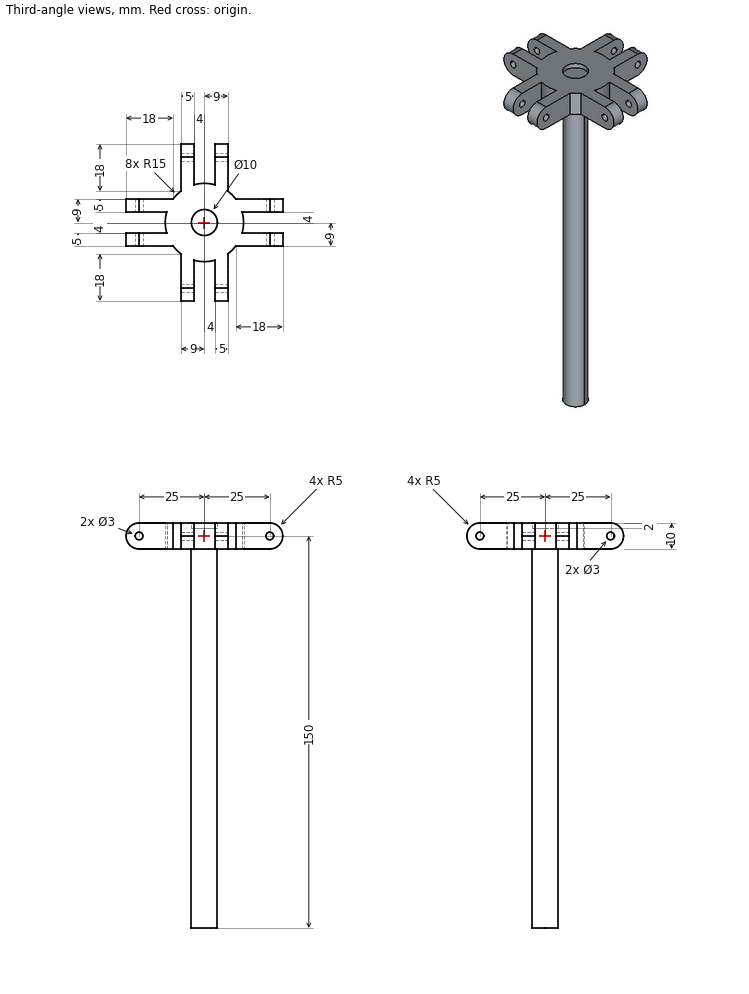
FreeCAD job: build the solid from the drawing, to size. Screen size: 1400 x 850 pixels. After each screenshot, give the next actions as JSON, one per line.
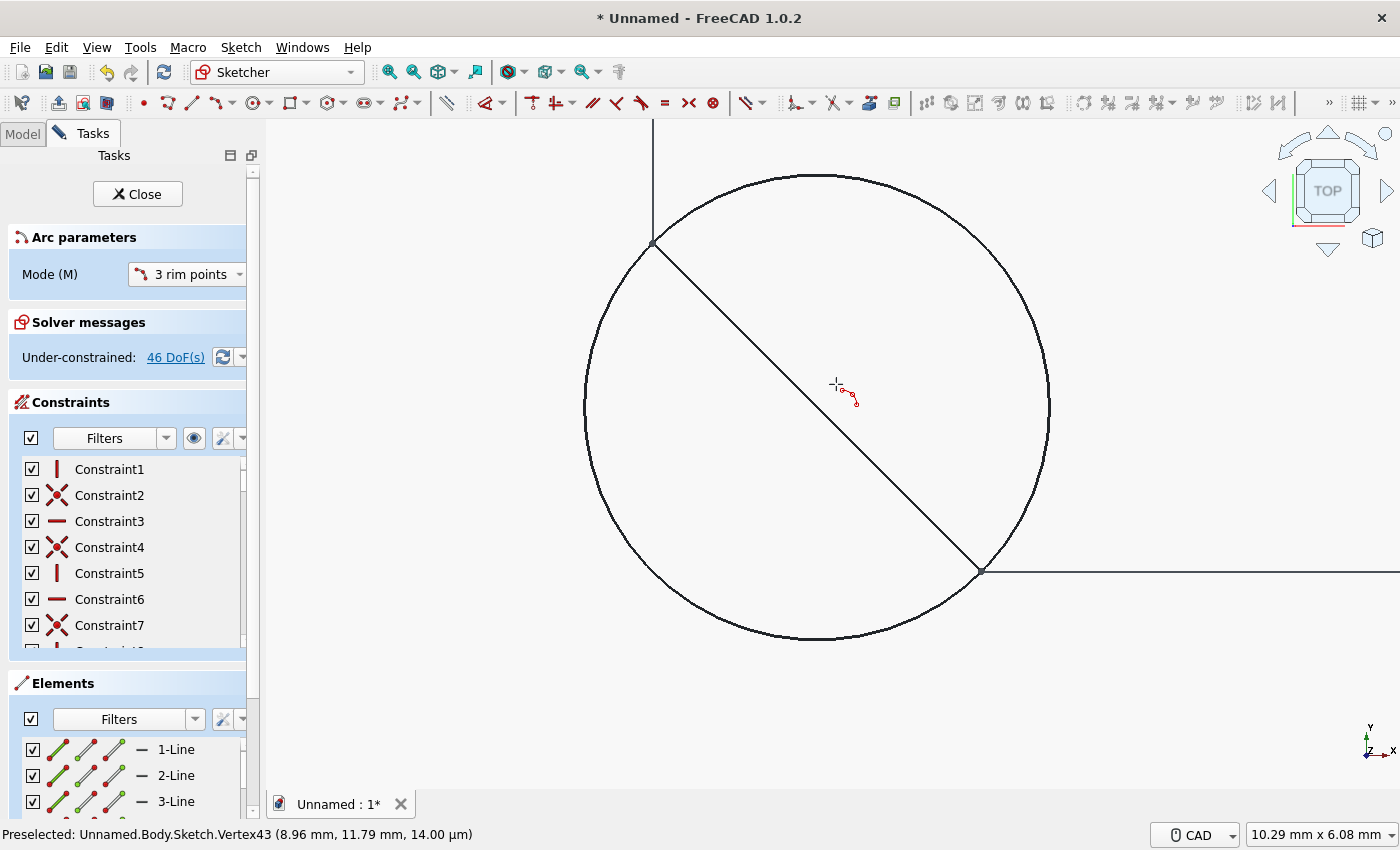
{"action": "left_click", "coordinate": [835, 374]}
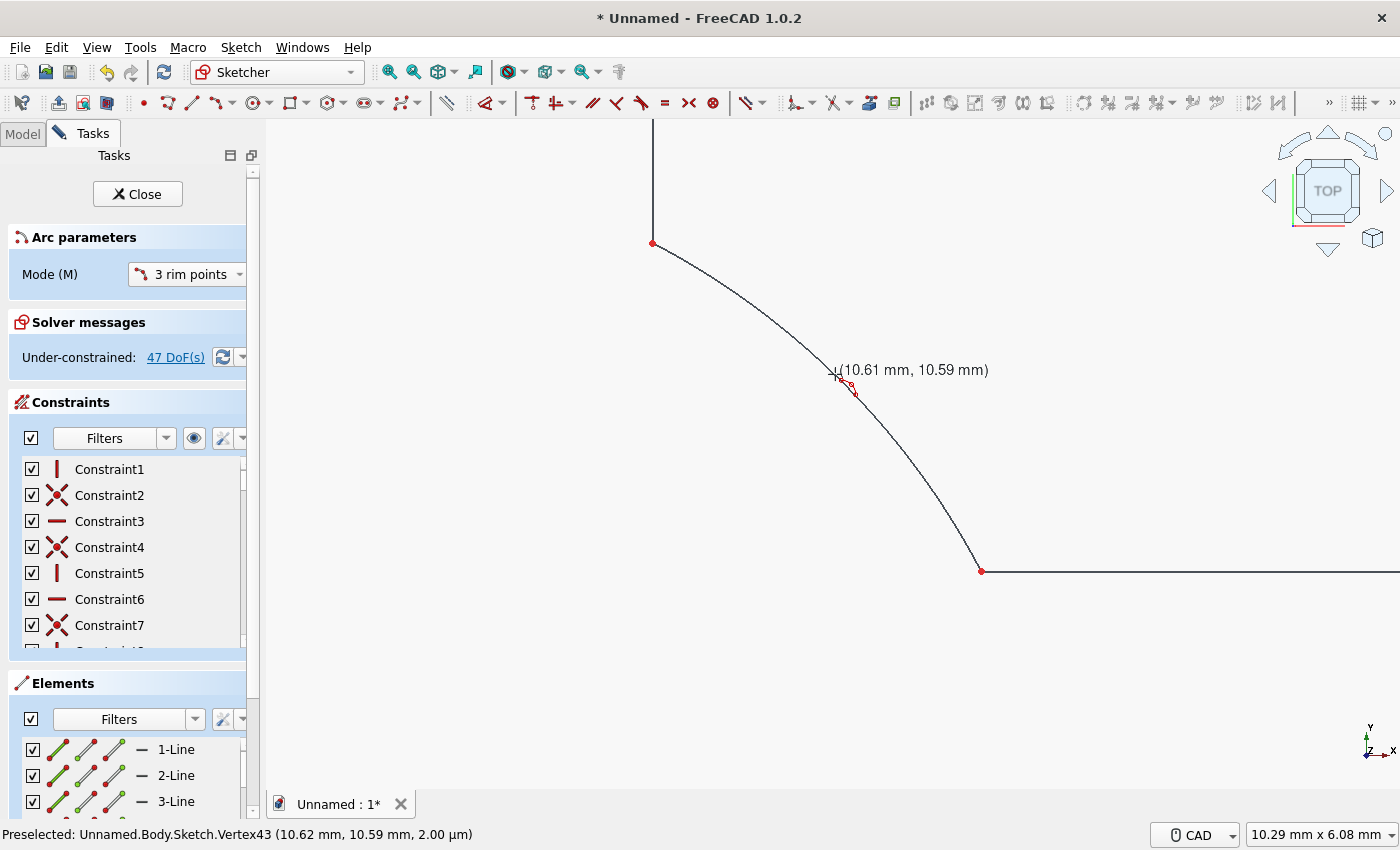
{"action": "scroll", "coordinate": [836, 384], "scroll_direction": "down", "scroll_amount": 14}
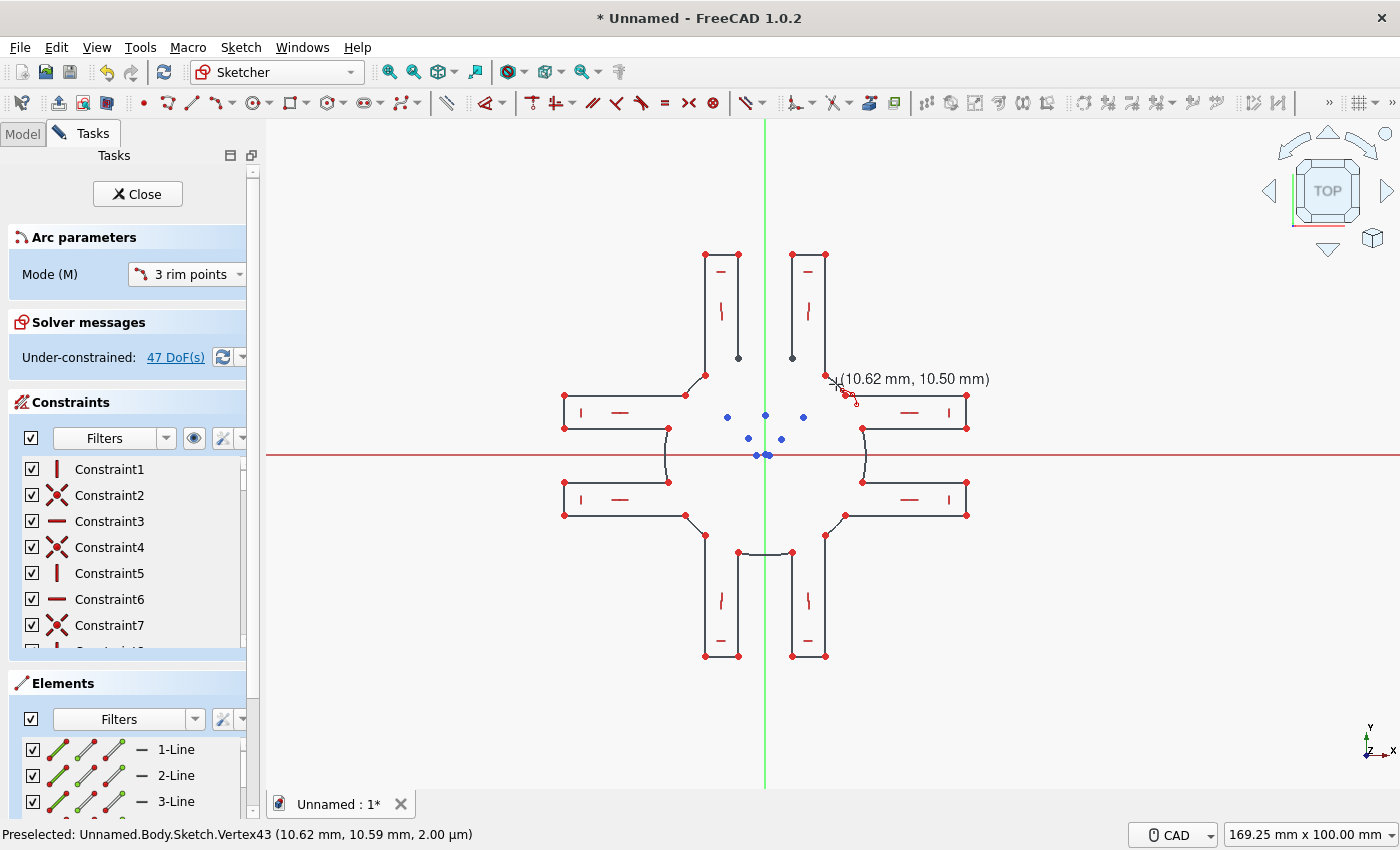
{"action": "left_click", "coordinate": [792, 359]}
{"action": "left_click", "coordinate": [738, 359]}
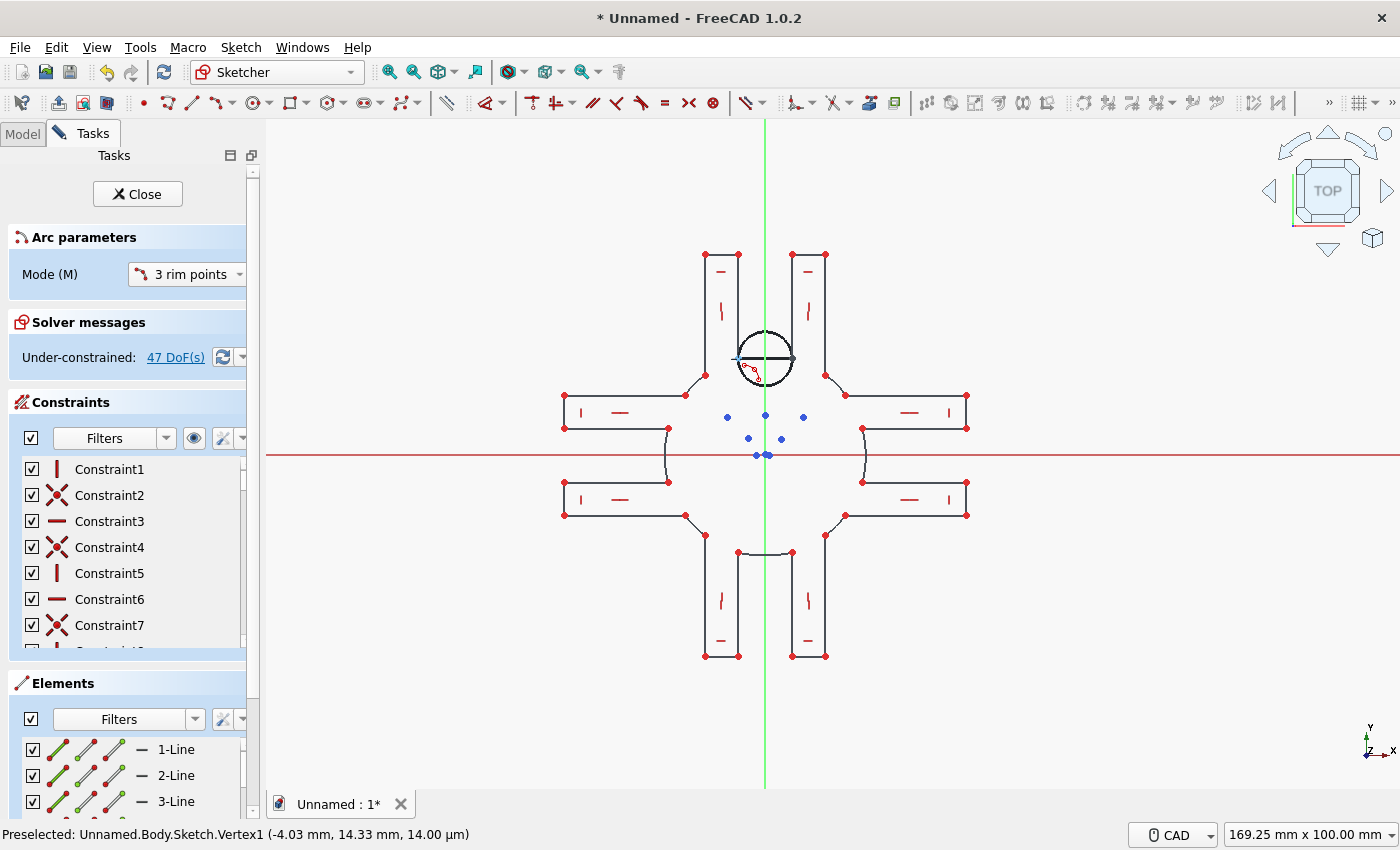
{"action": "scroll", "coordinate": [771, 354], "scroll_direction": "up", "scroll_amount": 8}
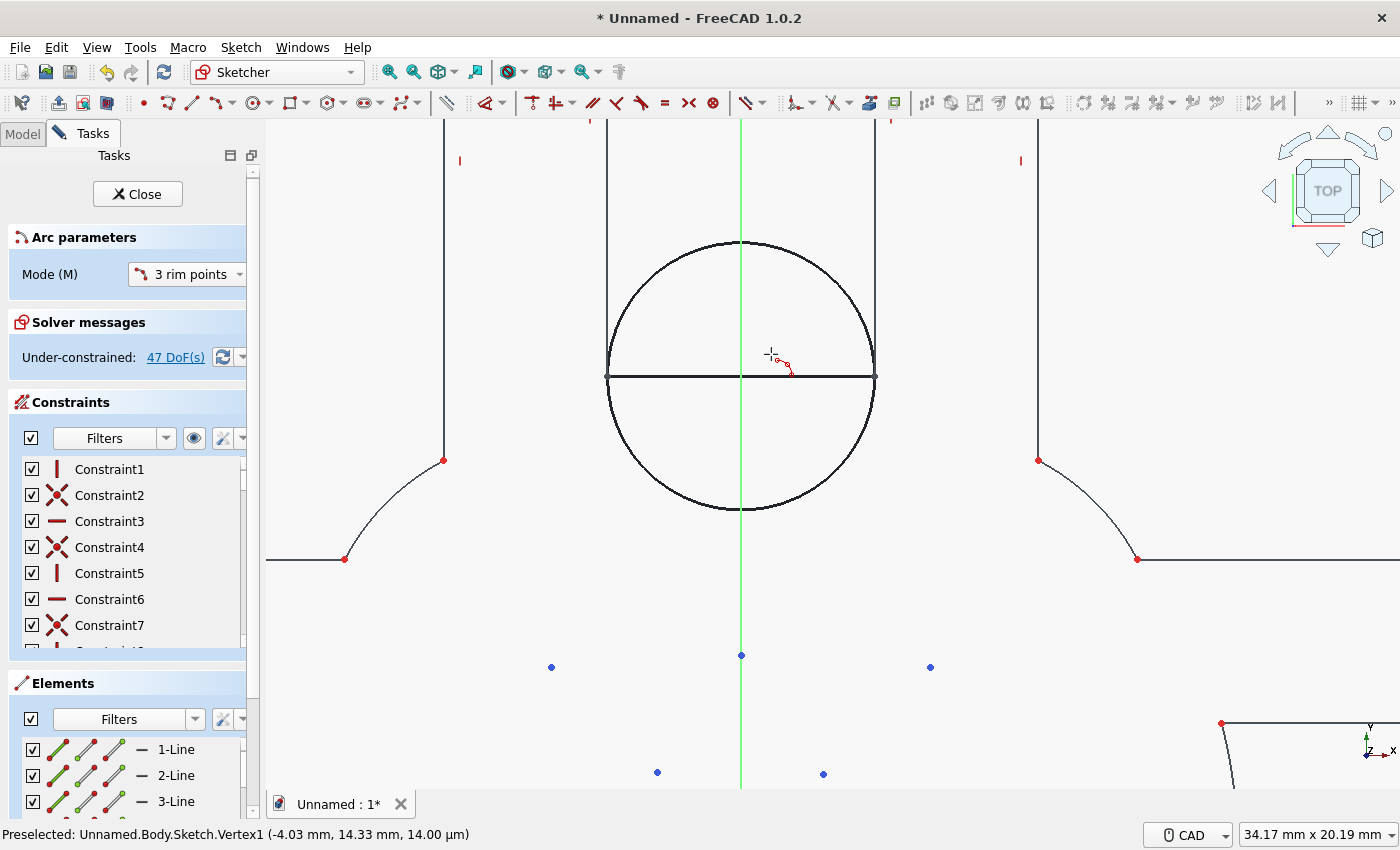
{"action": "left_click", "coordinate": [768, 355]}
{"action": "key", "text": "Escape"}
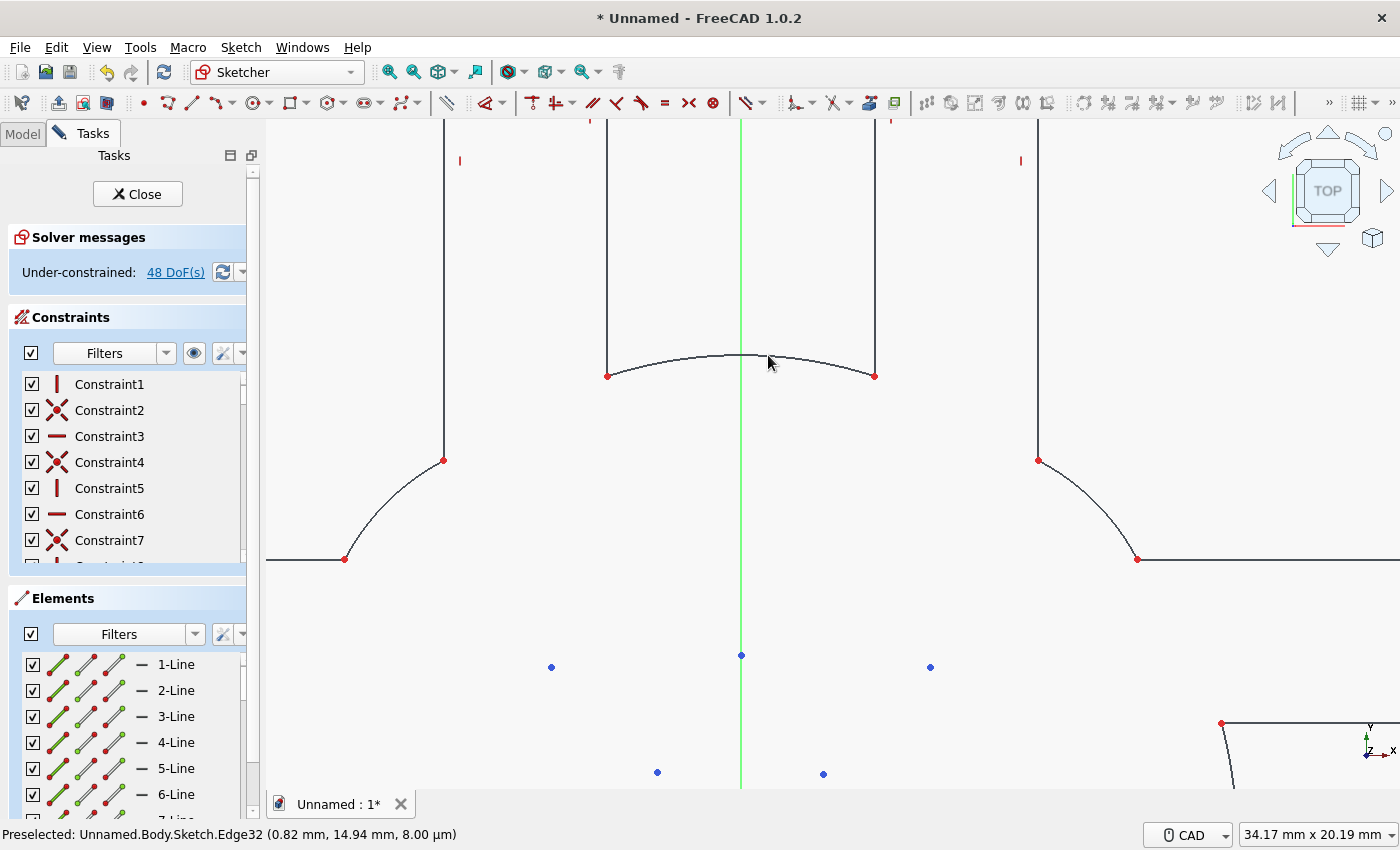
{"action": "scroll", "coordinate": [770, 353], "scroll_direction": "down", "scroll_amount": 8}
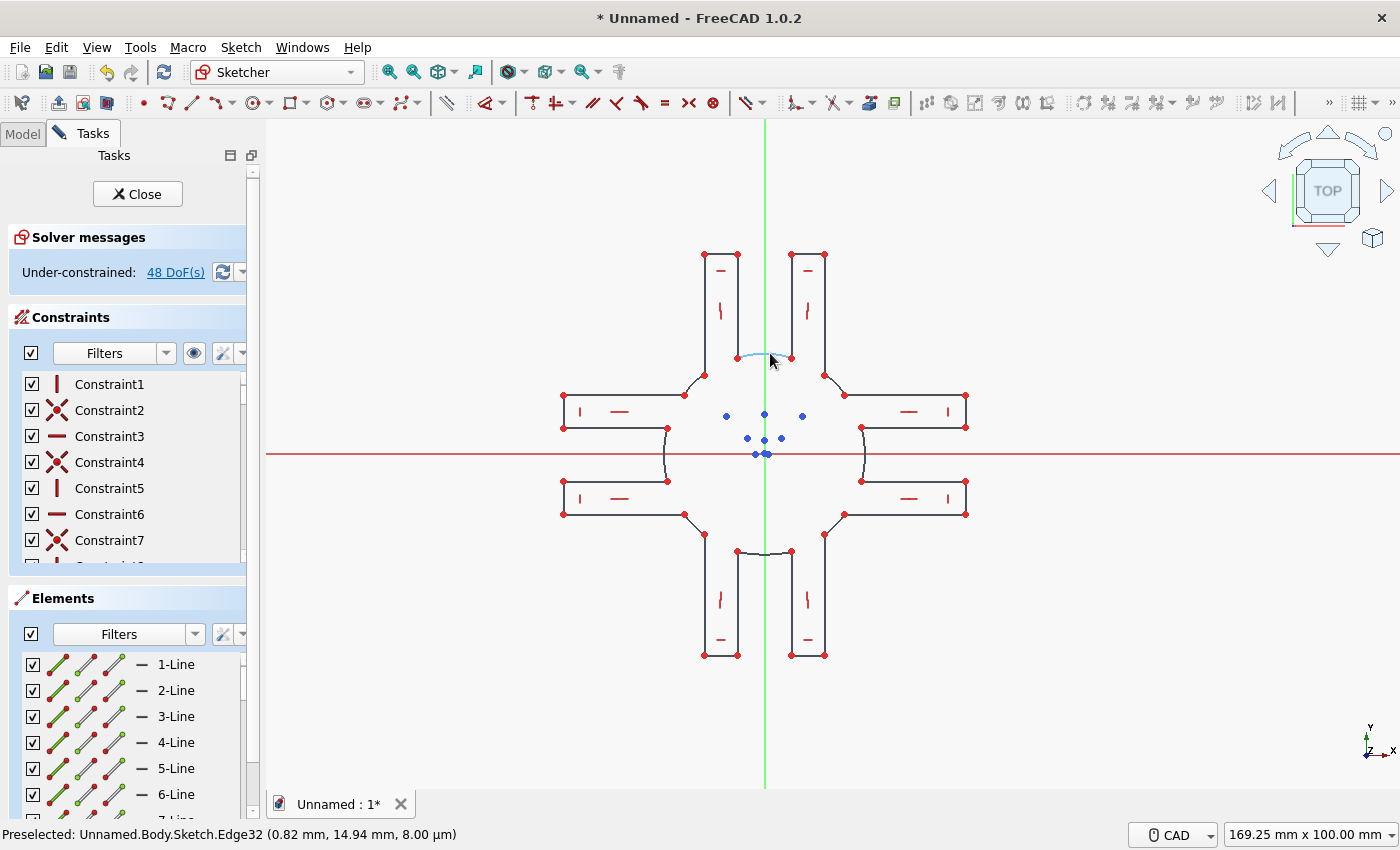
{"action": "scroll", "coordinate": [697, 380], "scroll_direction": "up", "scroll_amount": 3}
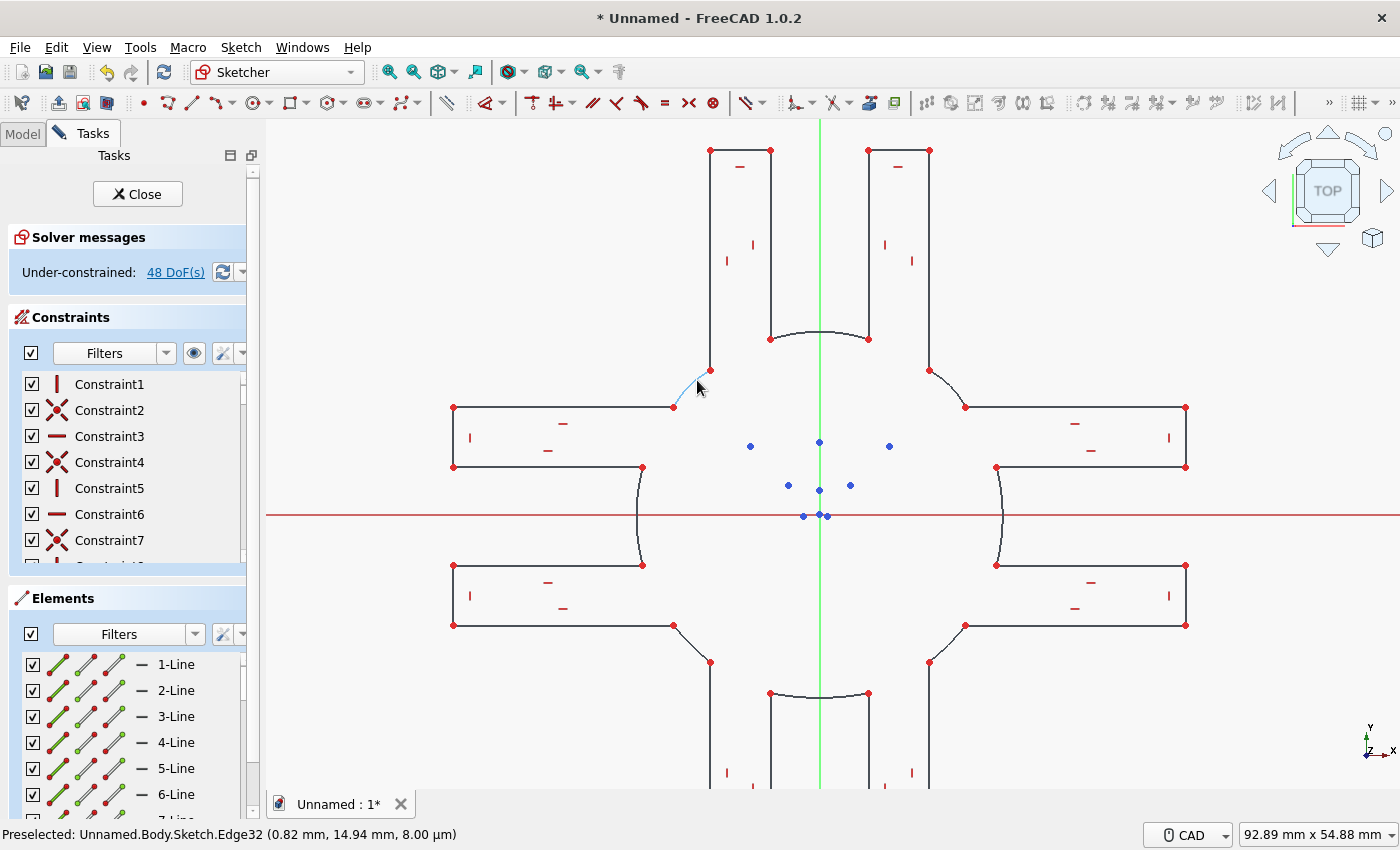
{"action": "left_click", "coordinate": [697, 379]}